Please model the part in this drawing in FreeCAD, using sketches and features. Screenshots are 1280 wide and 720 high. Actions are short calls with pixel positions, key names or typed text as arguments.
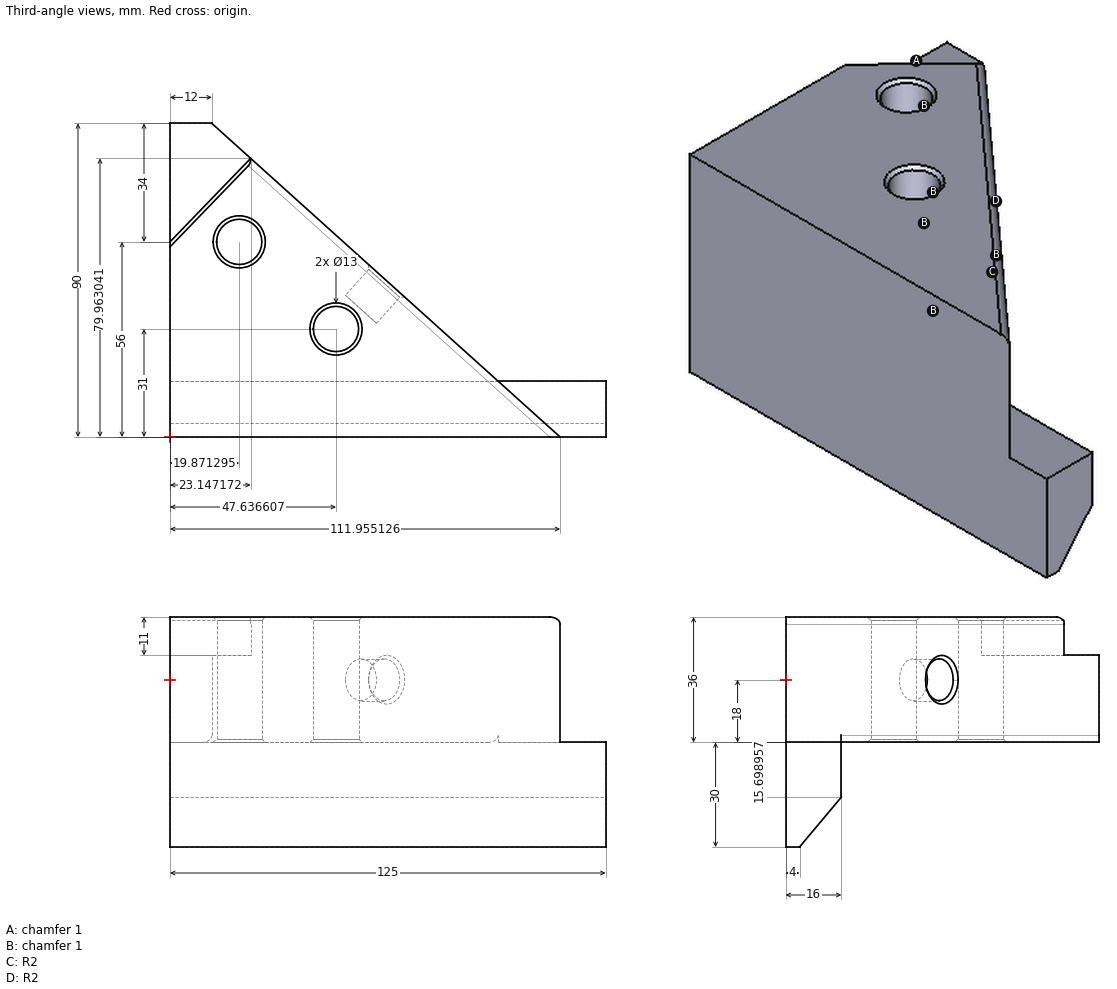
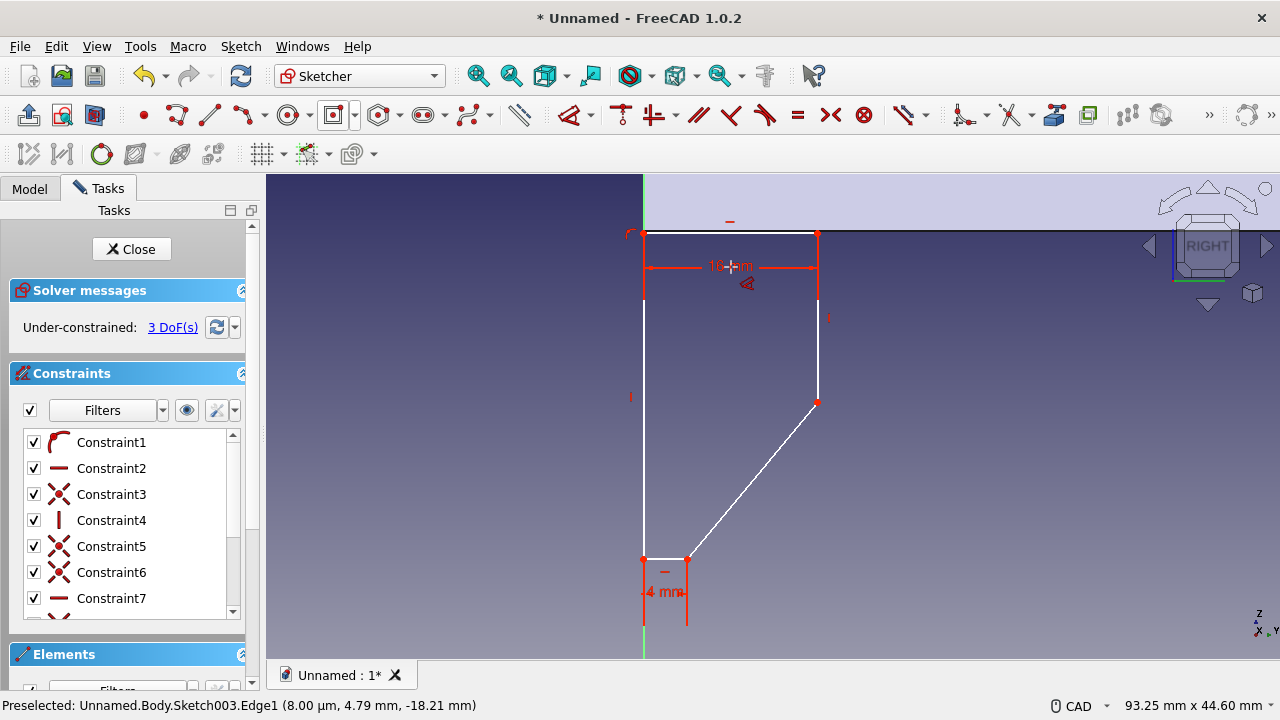
click(644, 461)
click(610, 396)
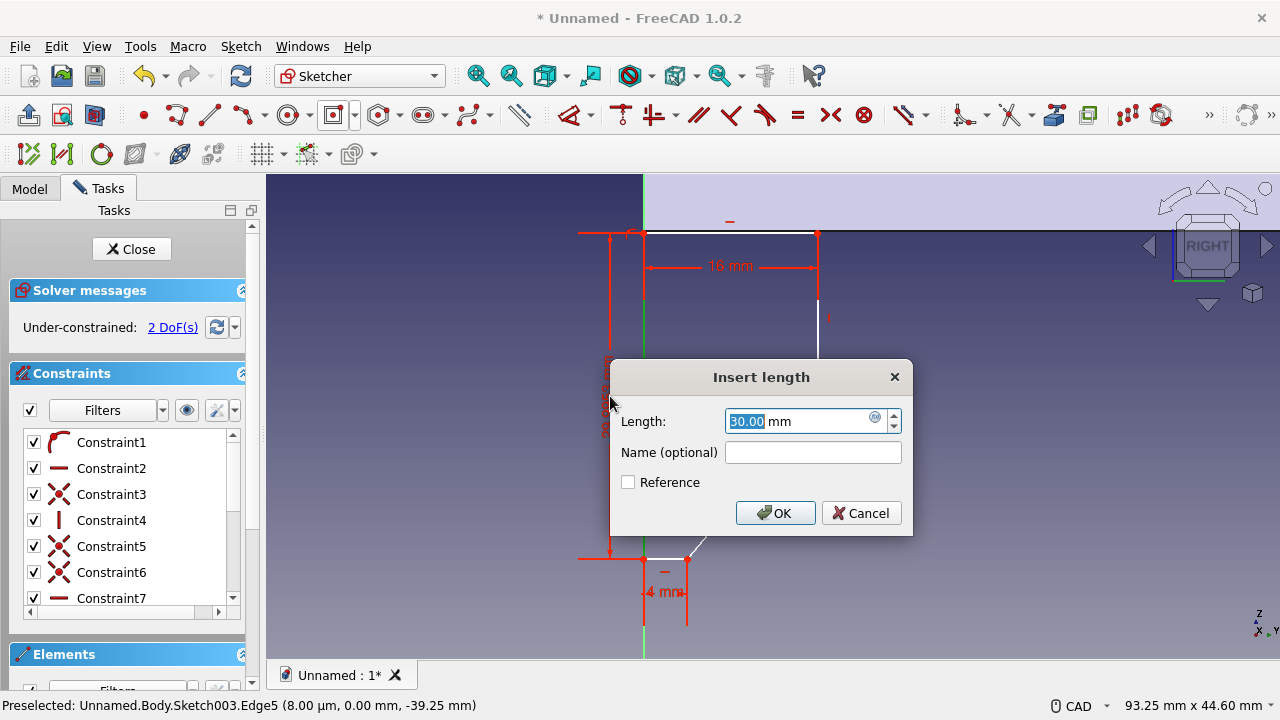
text(30)
key(Return)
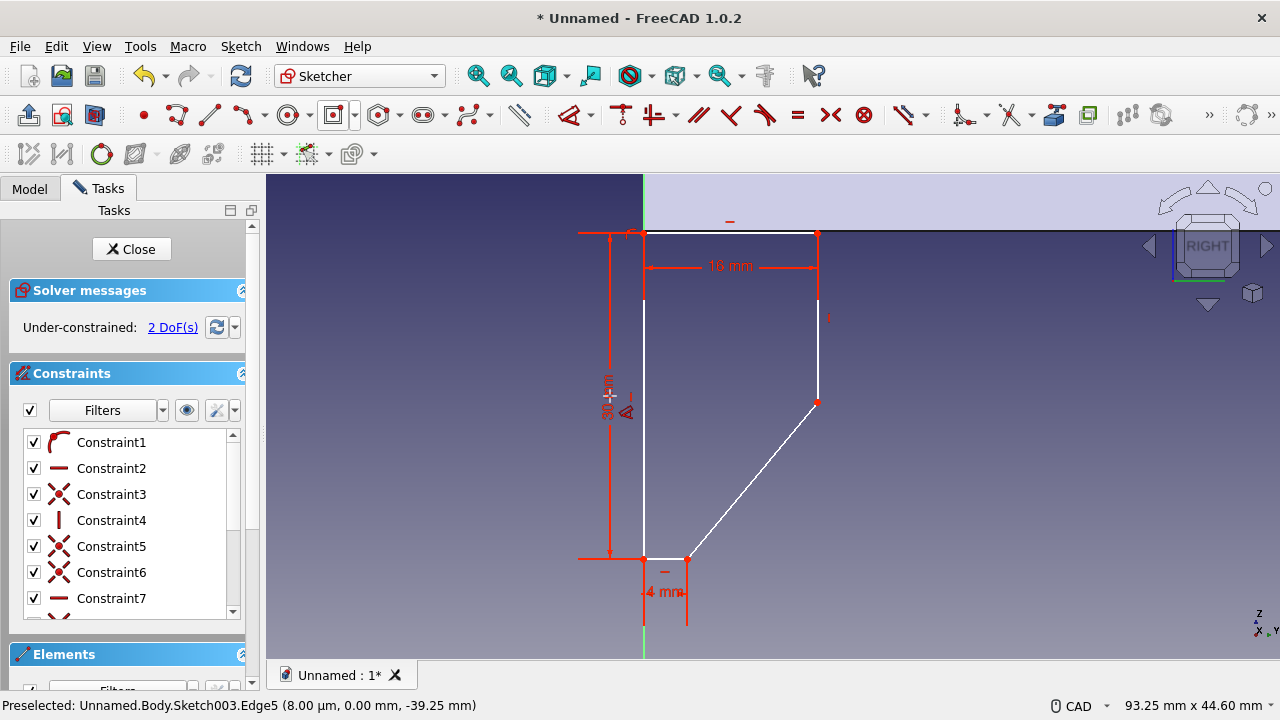
click(644, 233)
click(610, 218)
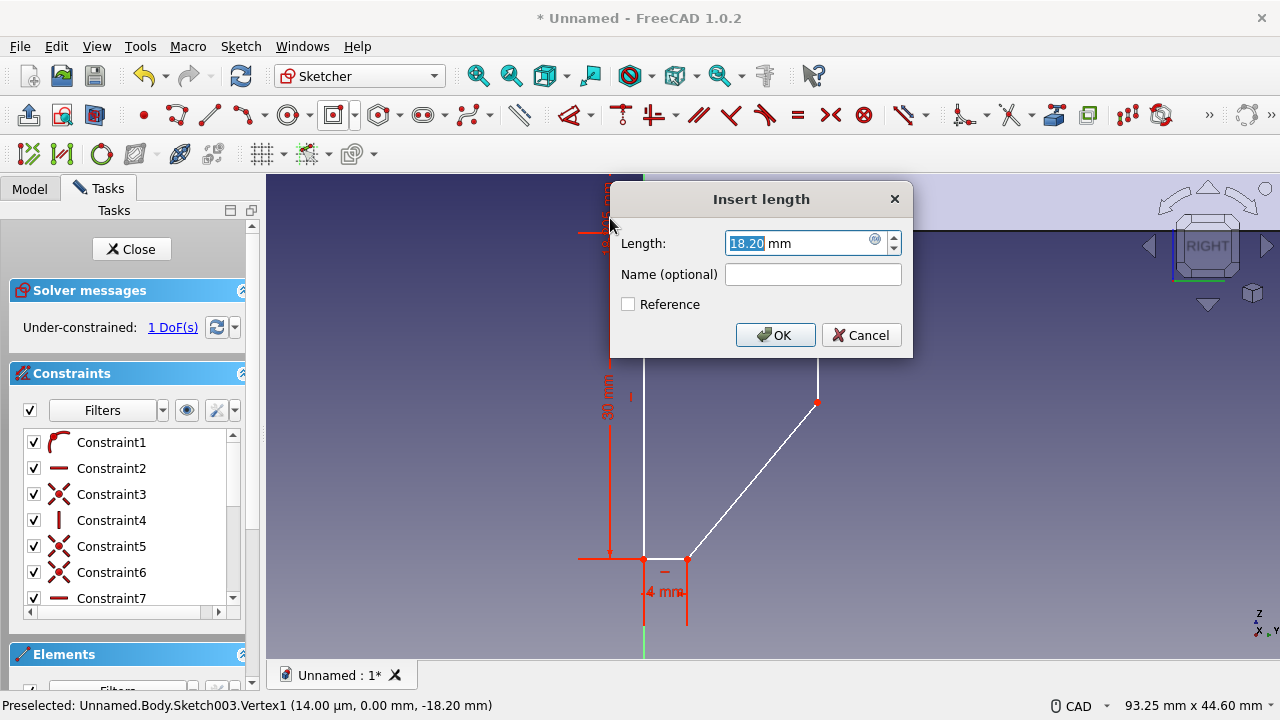
text(18)
key(Return)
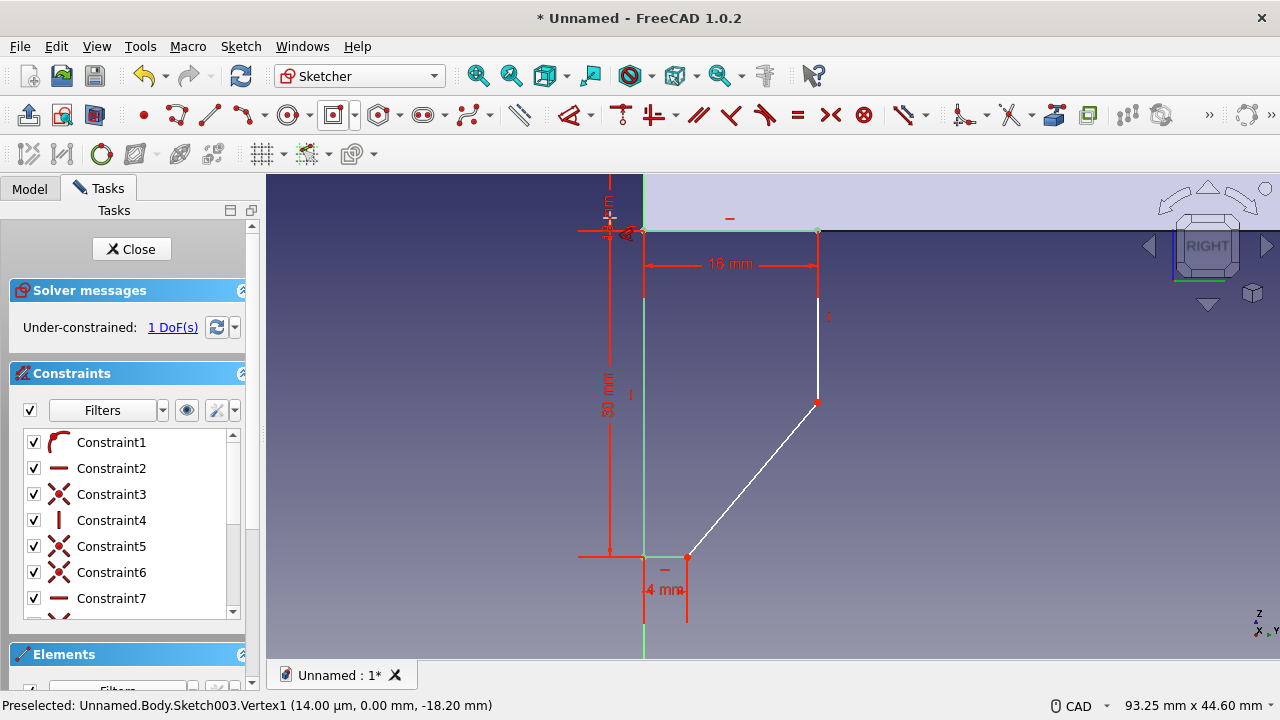
click(818, 282)
click(852, 317)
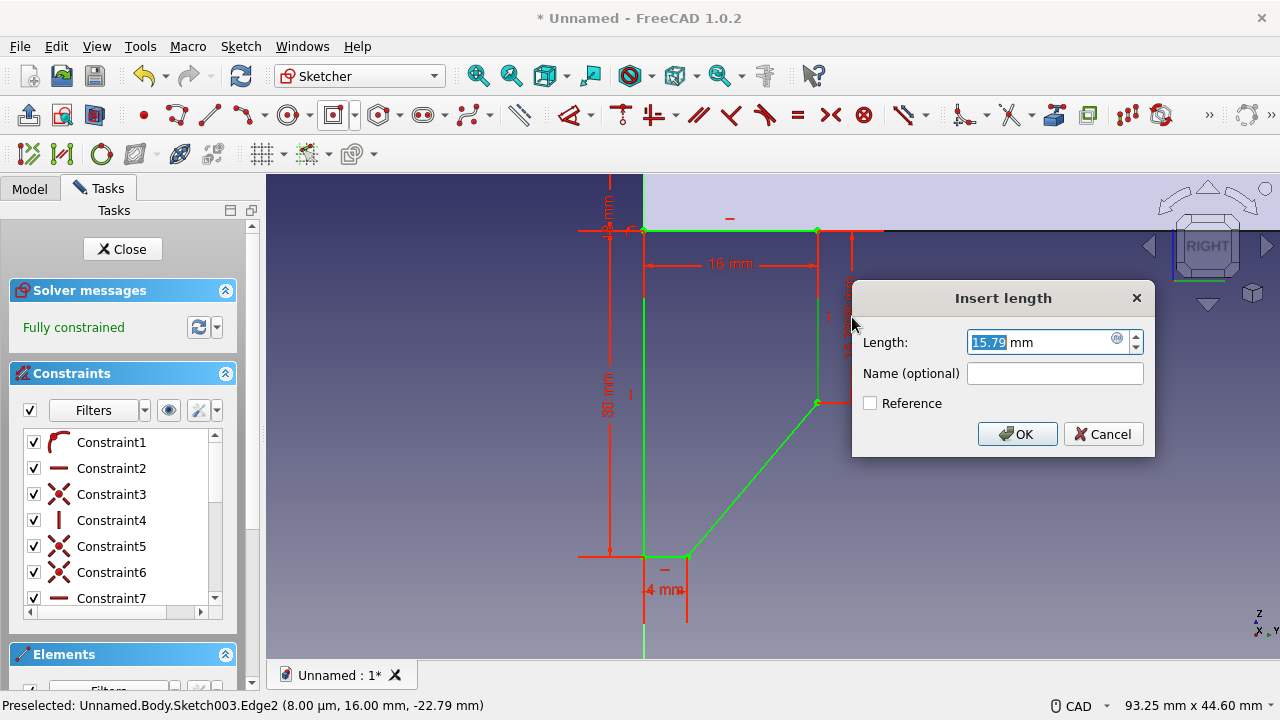
text(15.698957)
key(Return)
key(Escape)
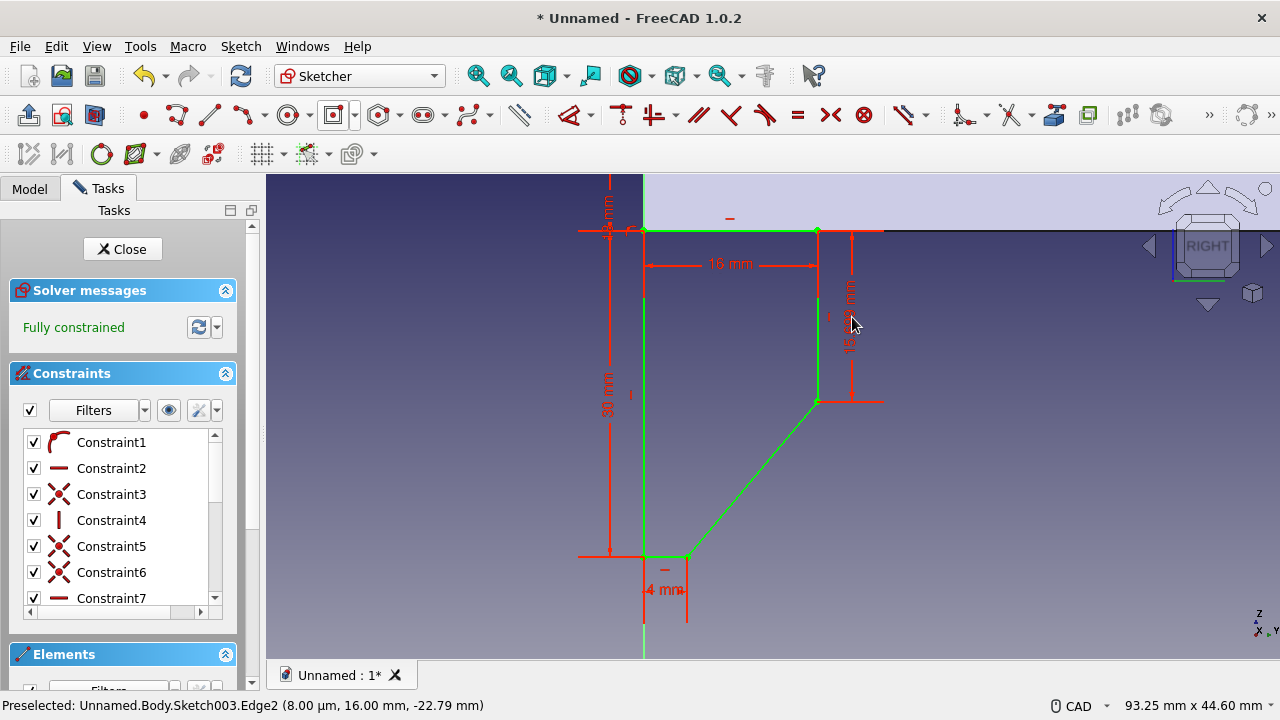
click(123, 249)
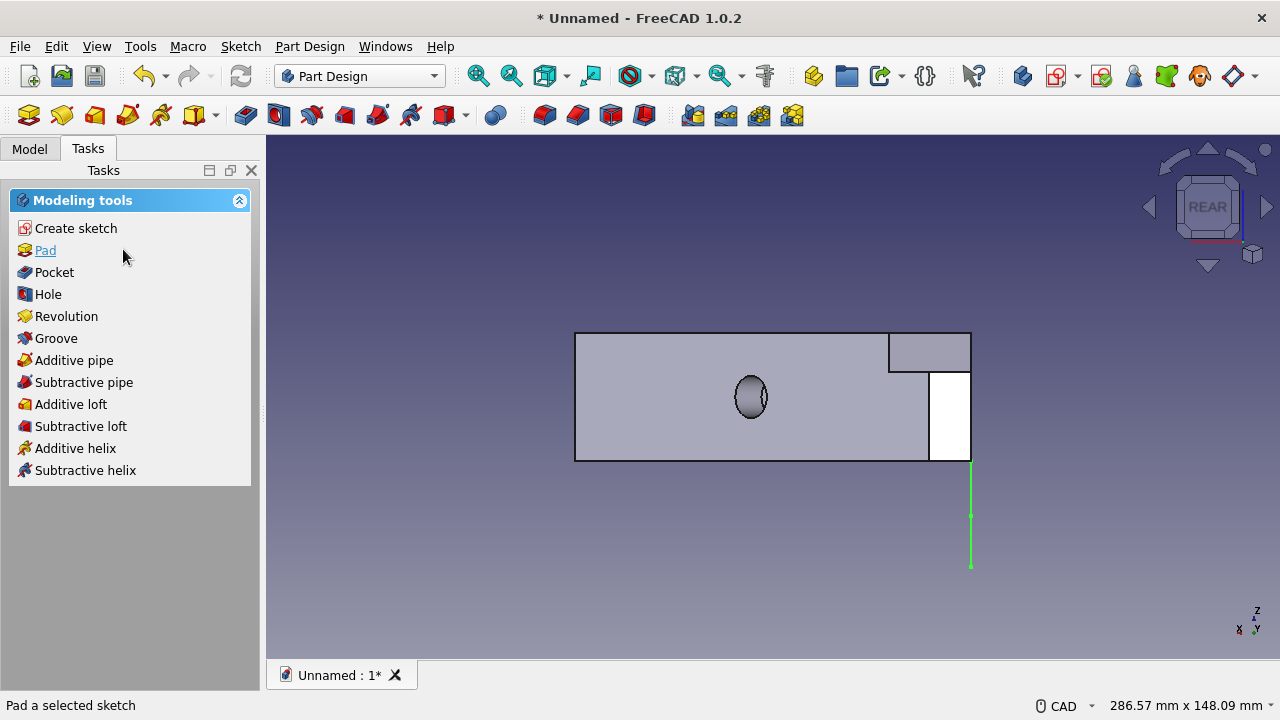
click(29, 116)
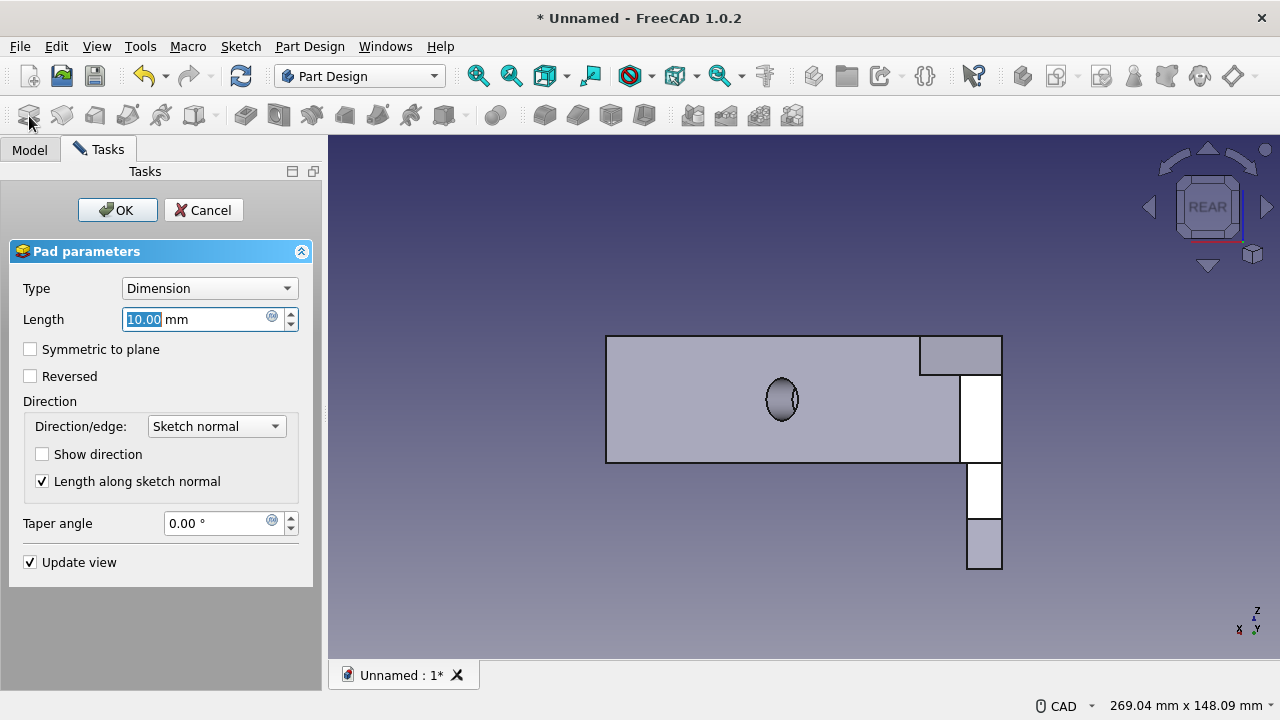
text(125)
key(Tab)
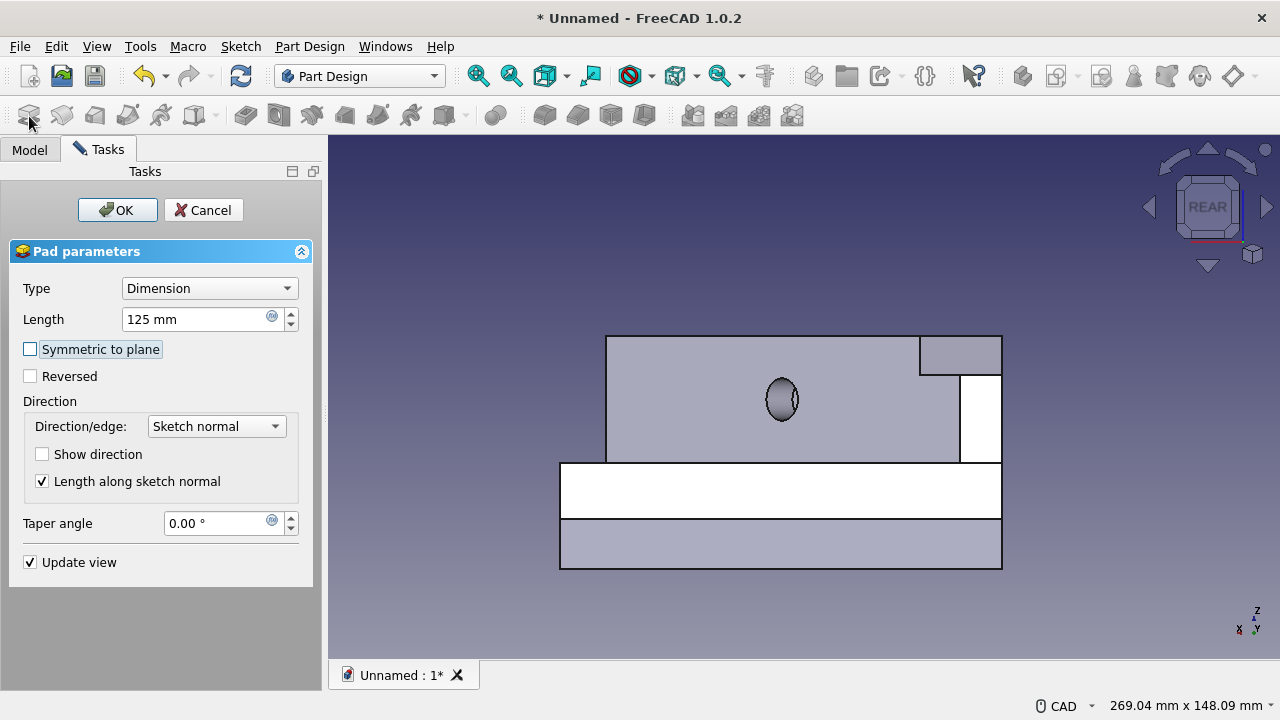
click(118, 210)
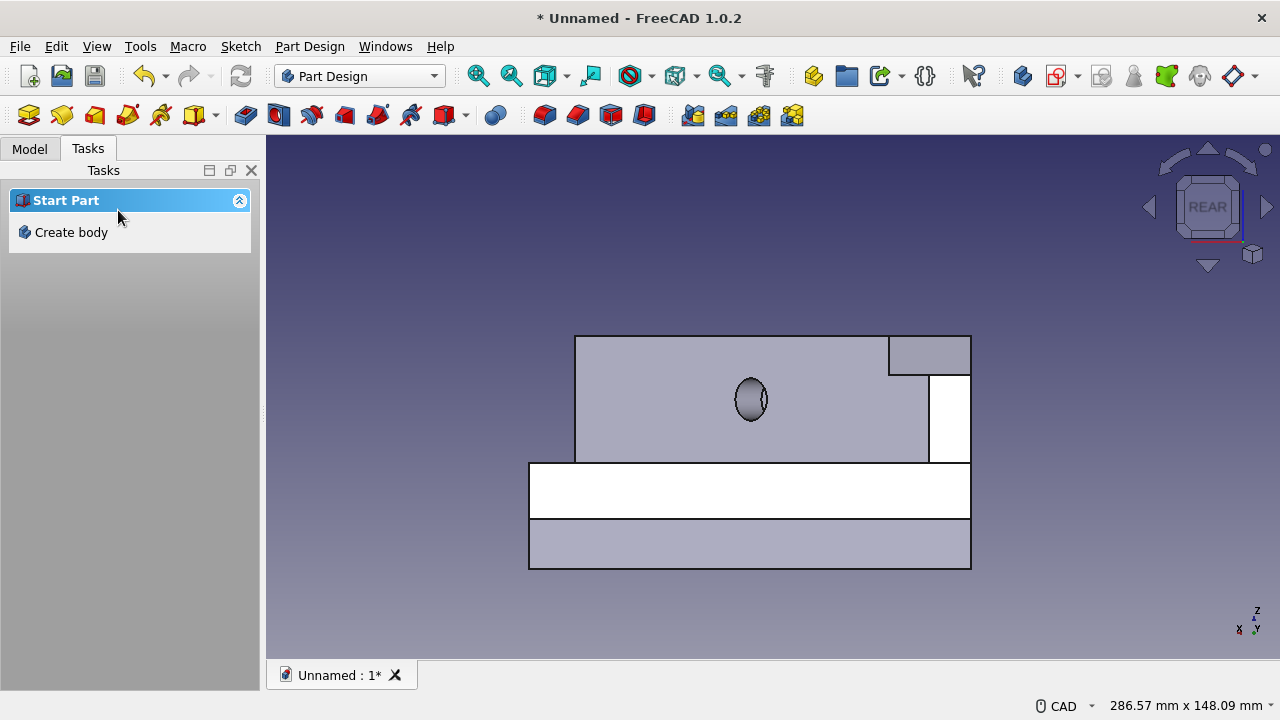
click(479, 76)